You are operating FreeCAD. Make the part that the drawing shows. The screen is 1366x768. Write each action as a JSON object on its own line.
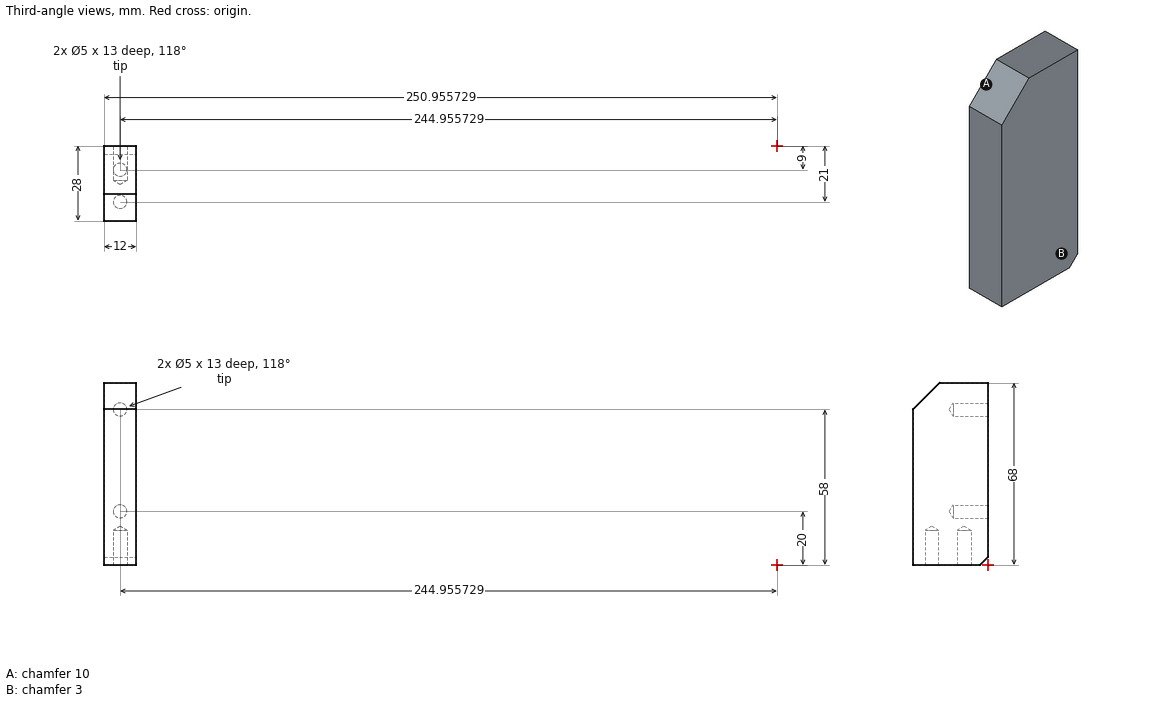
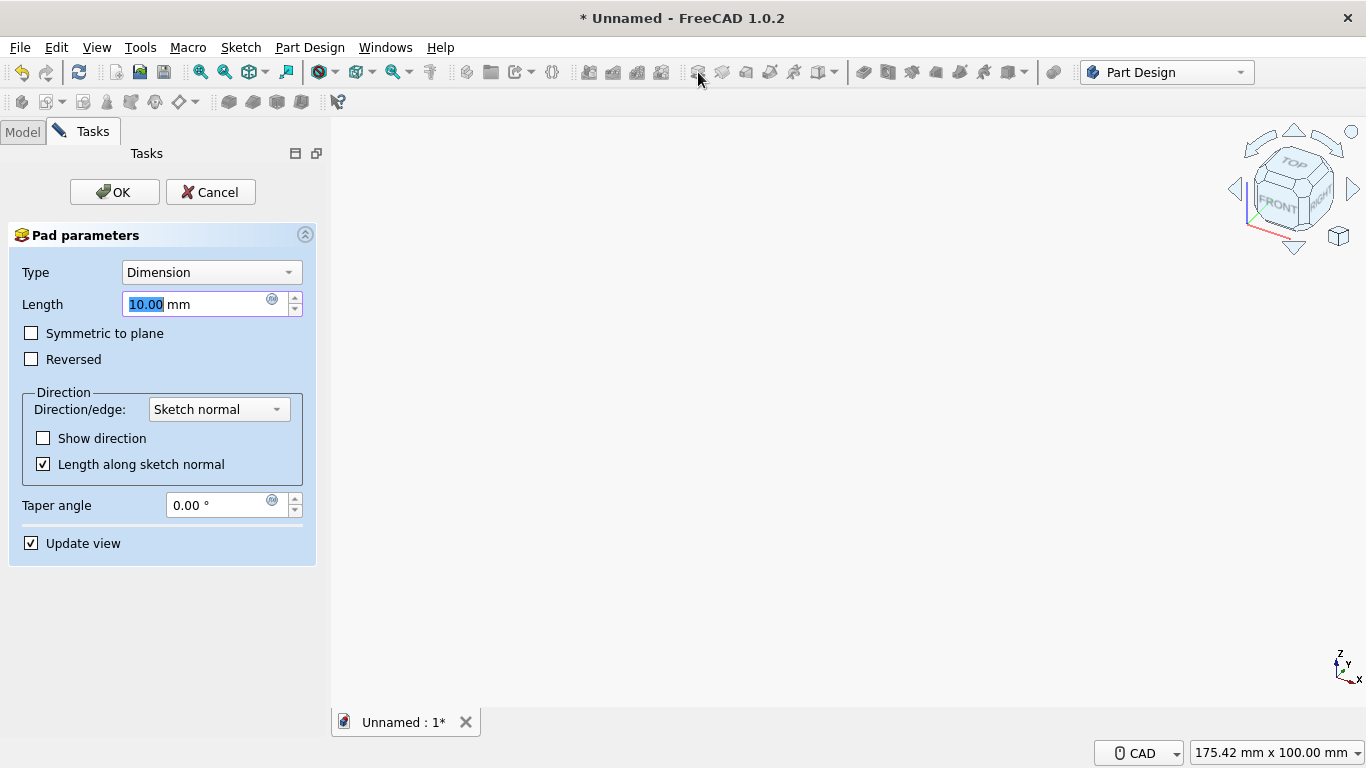
{"action": "type", "text": "68"}
{"action": "key", "text": "Tab"}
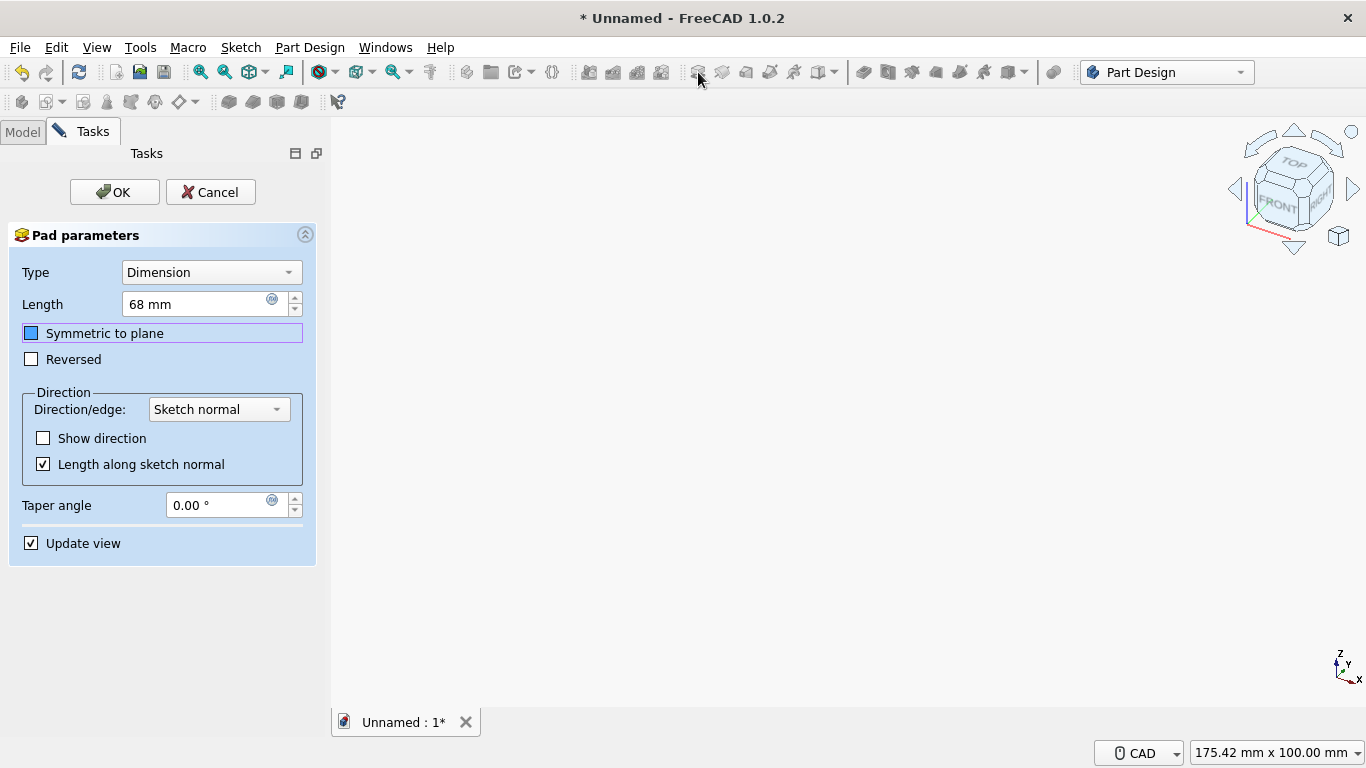
{"action": "left_click", "coordinate": [115, 192]}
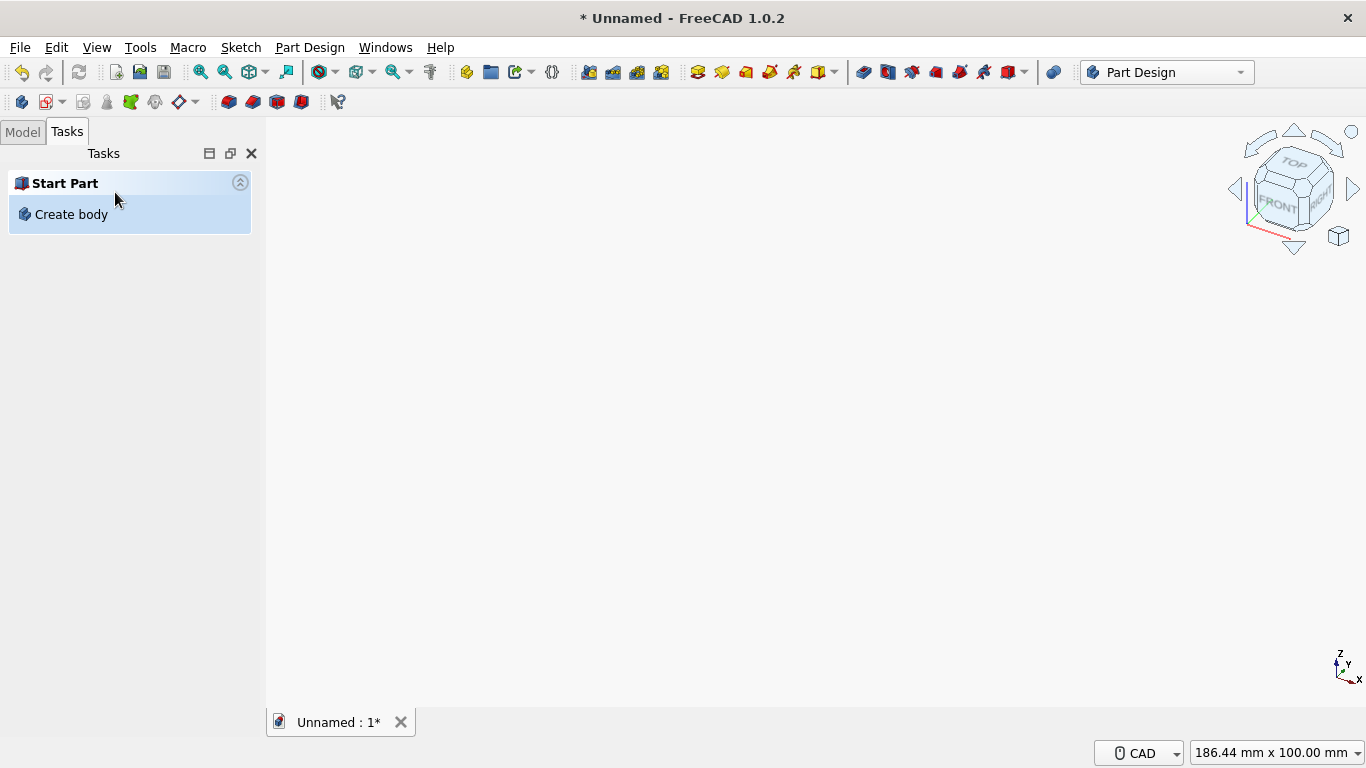
{"action": "left_click", "coordinate": [202, 72]}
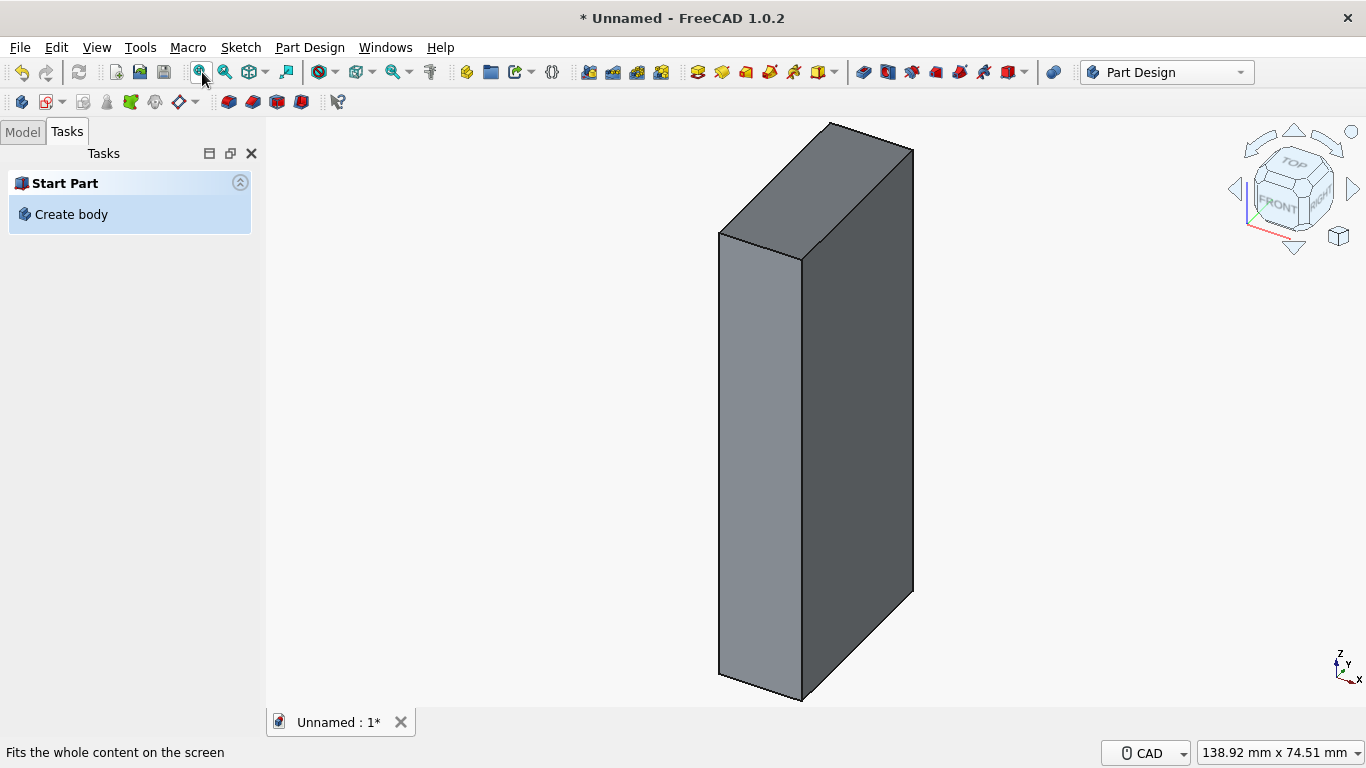
{"action": "left_click", "coordinate": [761, 246]}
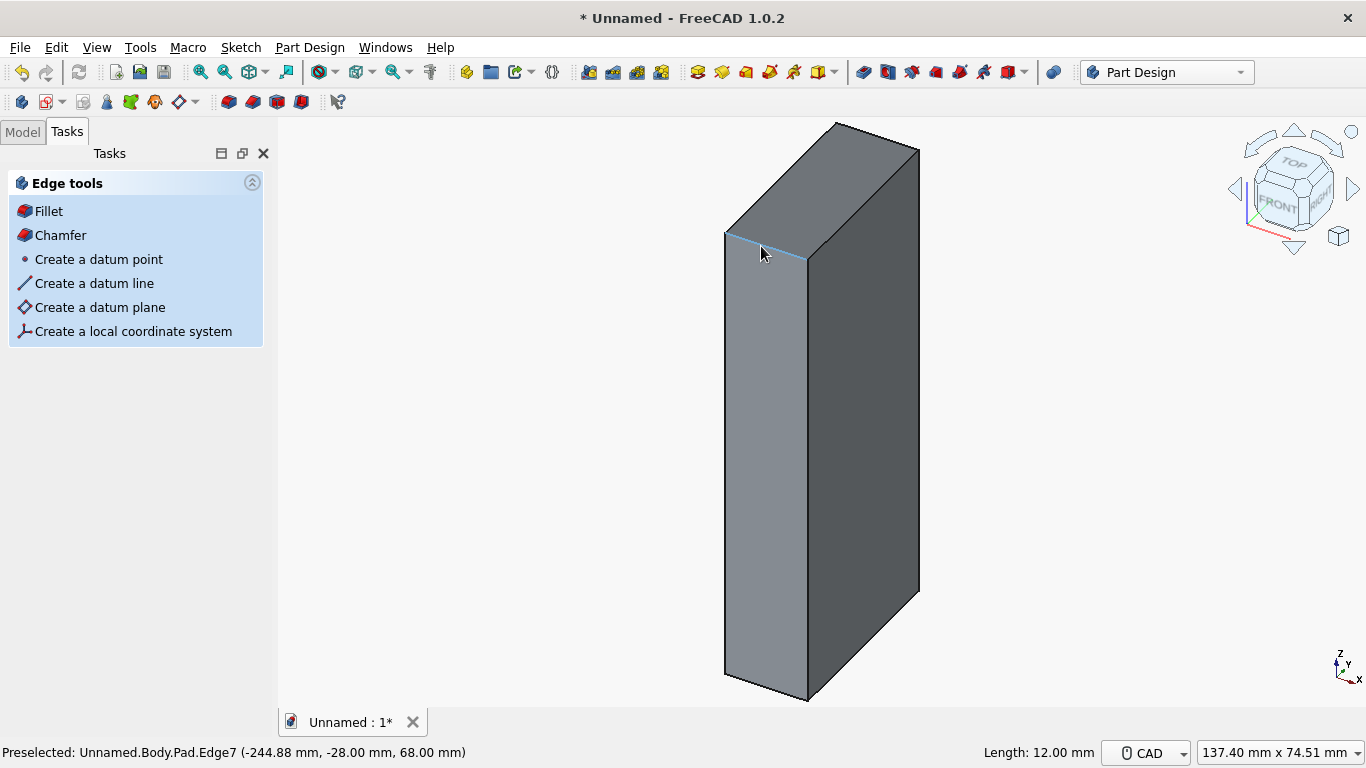
{"action": "left_click", "coordinate": [254, 102]}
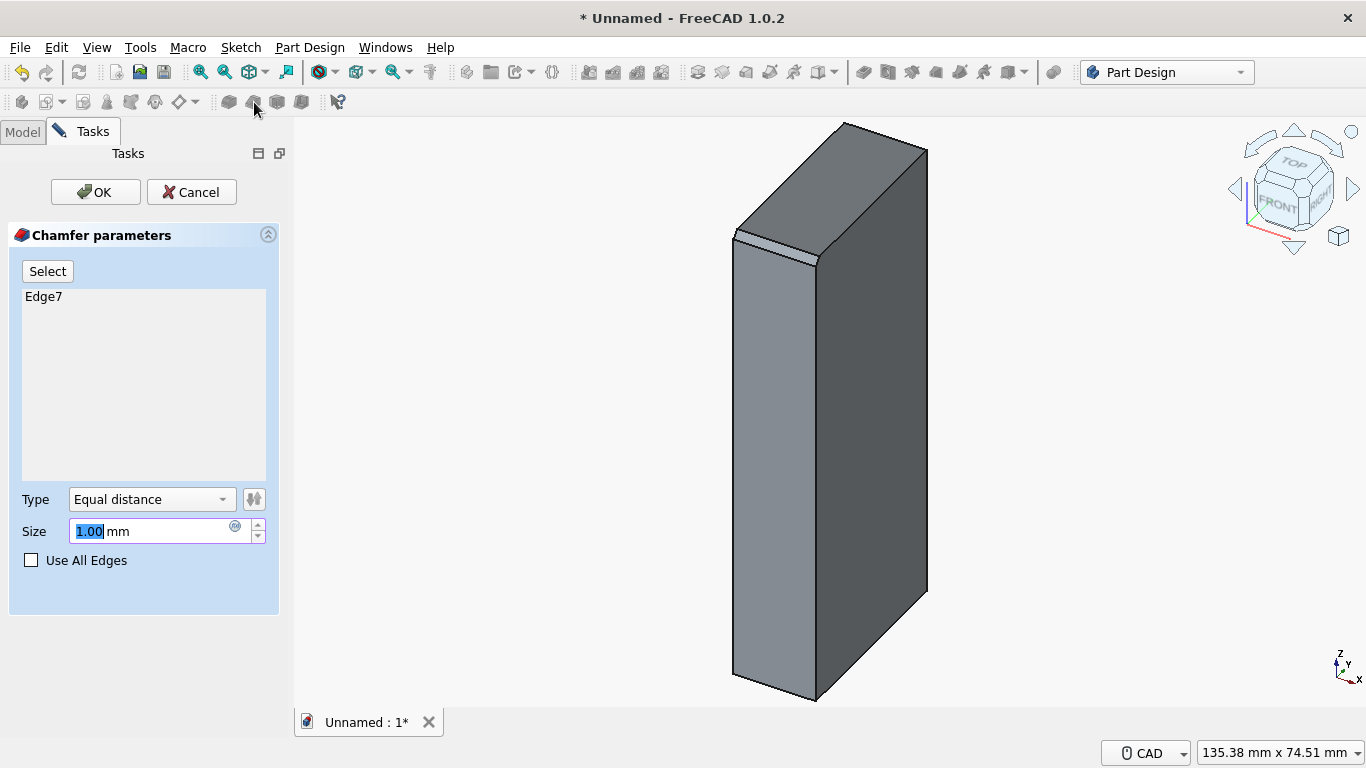
{"action": "type", "text": "10"}
{"action": "key", "text": "Tab"}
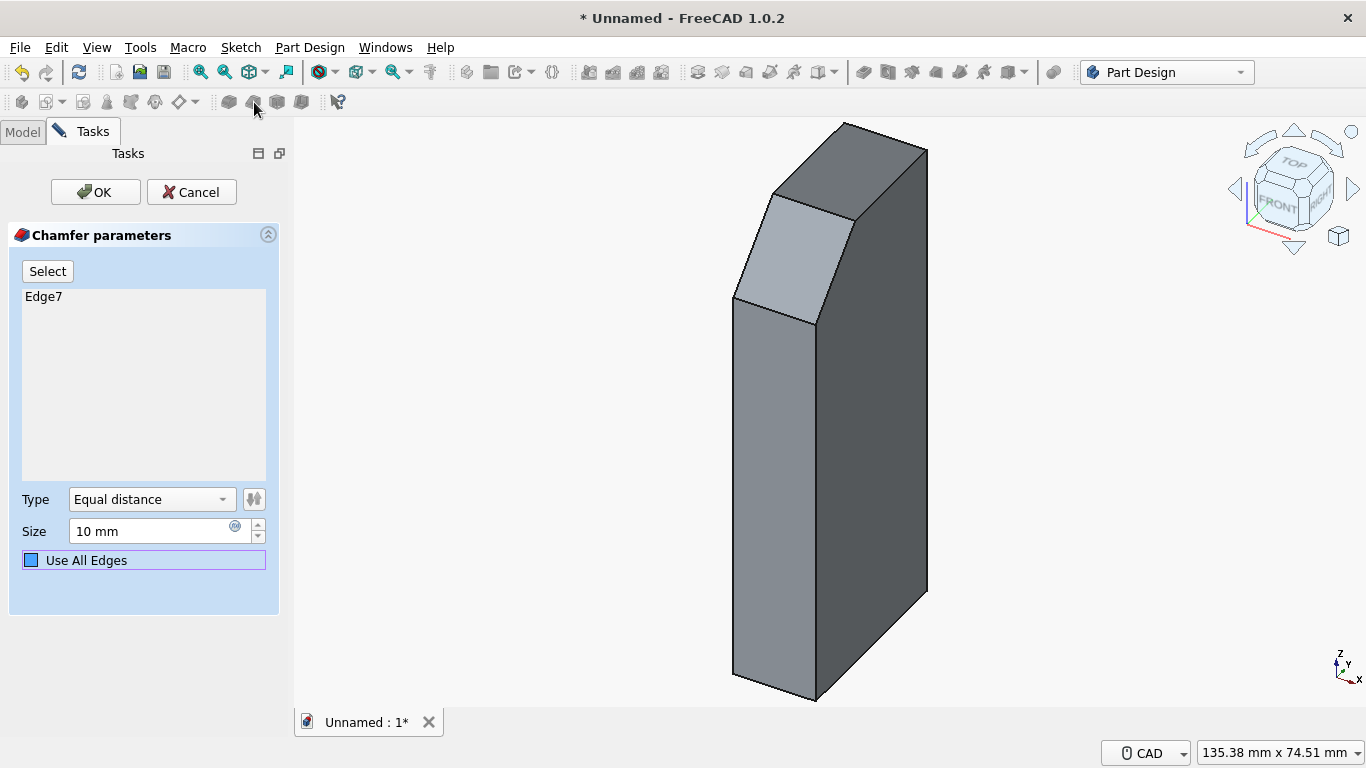
{"action": "left_click", "coordinate": [96, 192]}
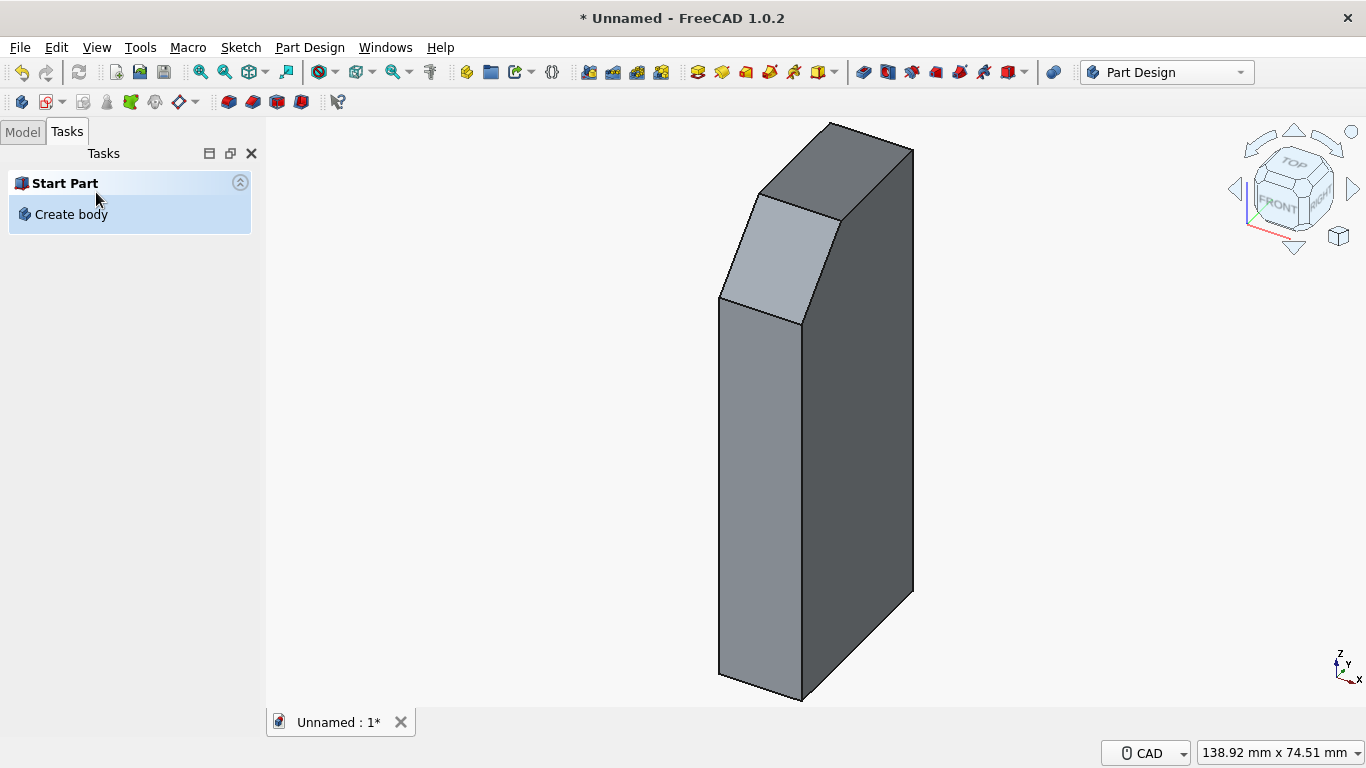
{"action": "key", "text": "0"}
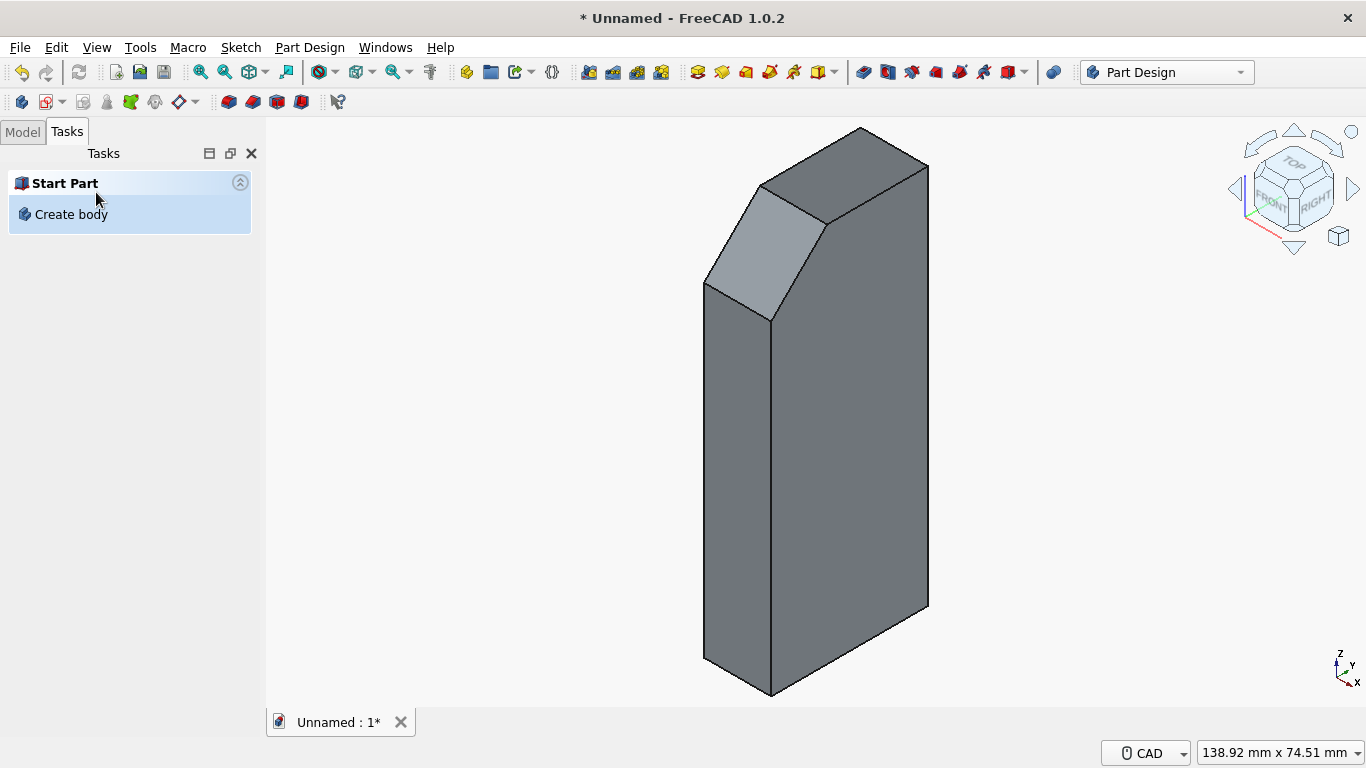
{"action": "key", "text": "2"}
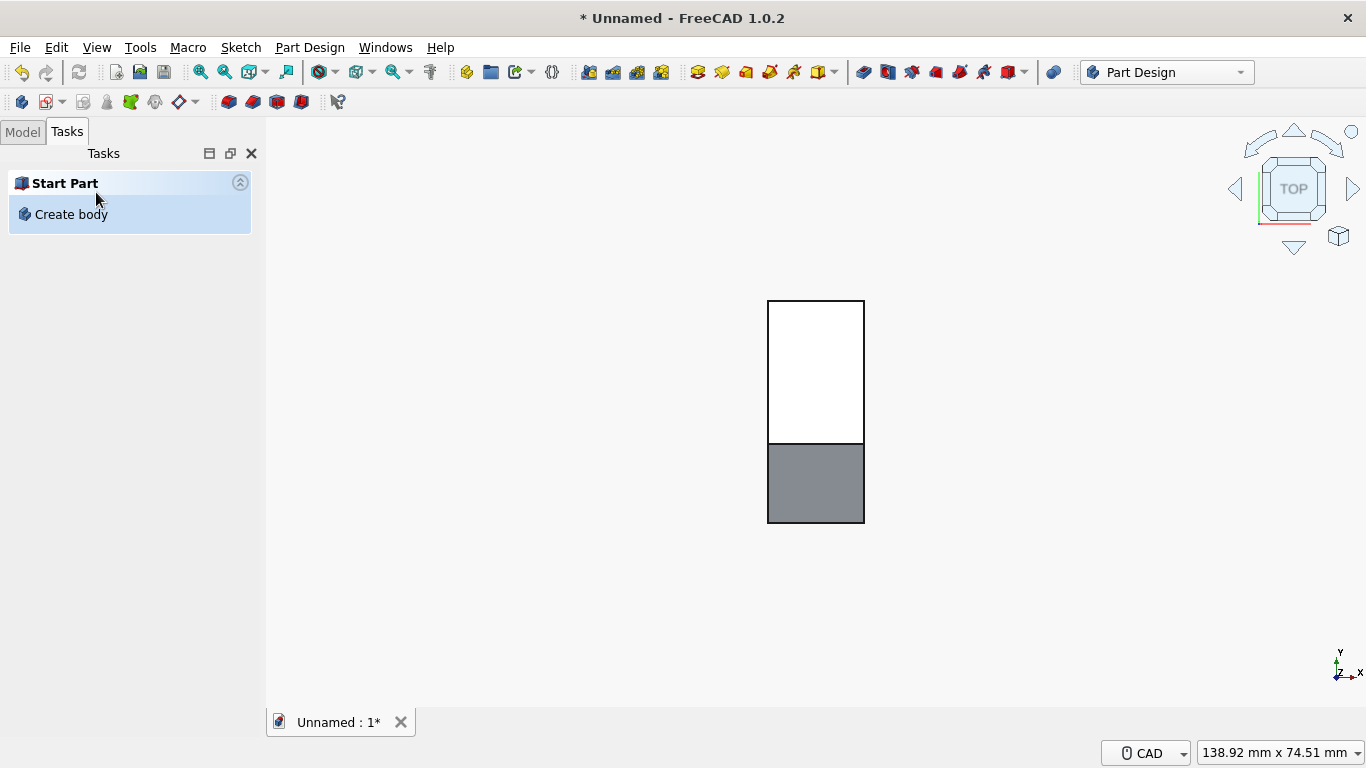
{"action": "left_click", "coordinate": [202, 72]}